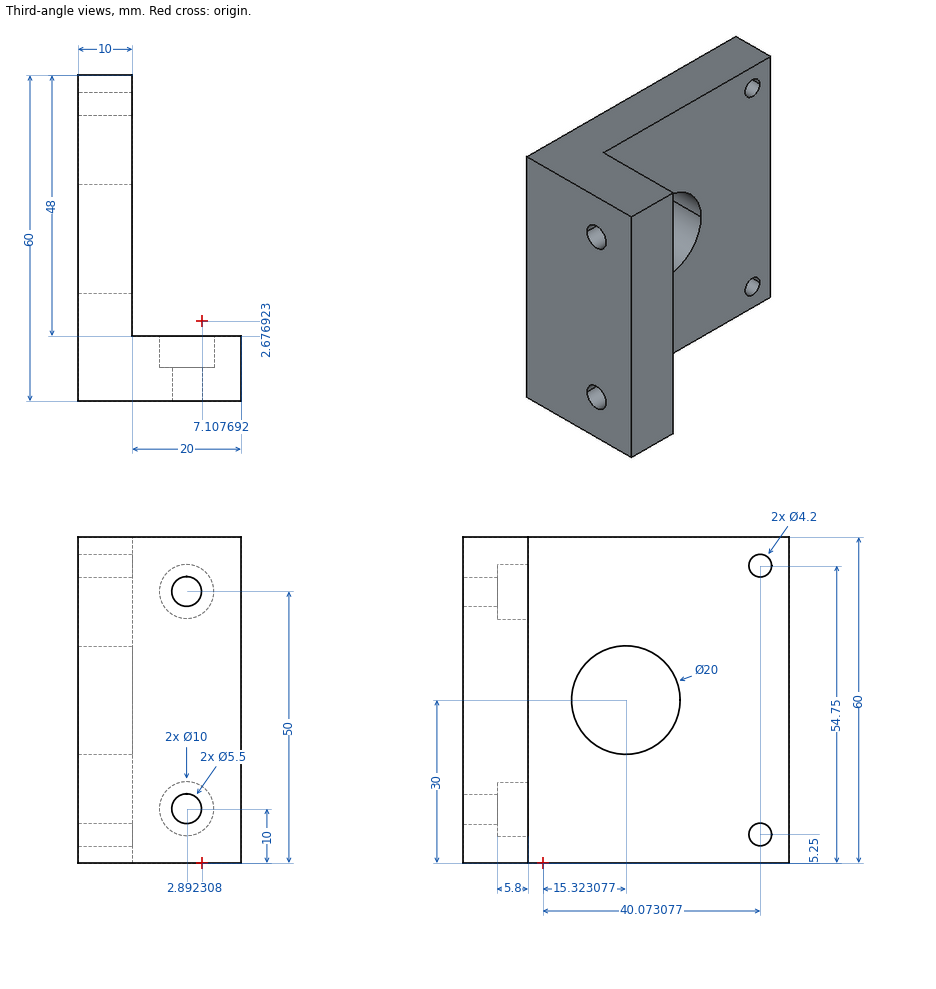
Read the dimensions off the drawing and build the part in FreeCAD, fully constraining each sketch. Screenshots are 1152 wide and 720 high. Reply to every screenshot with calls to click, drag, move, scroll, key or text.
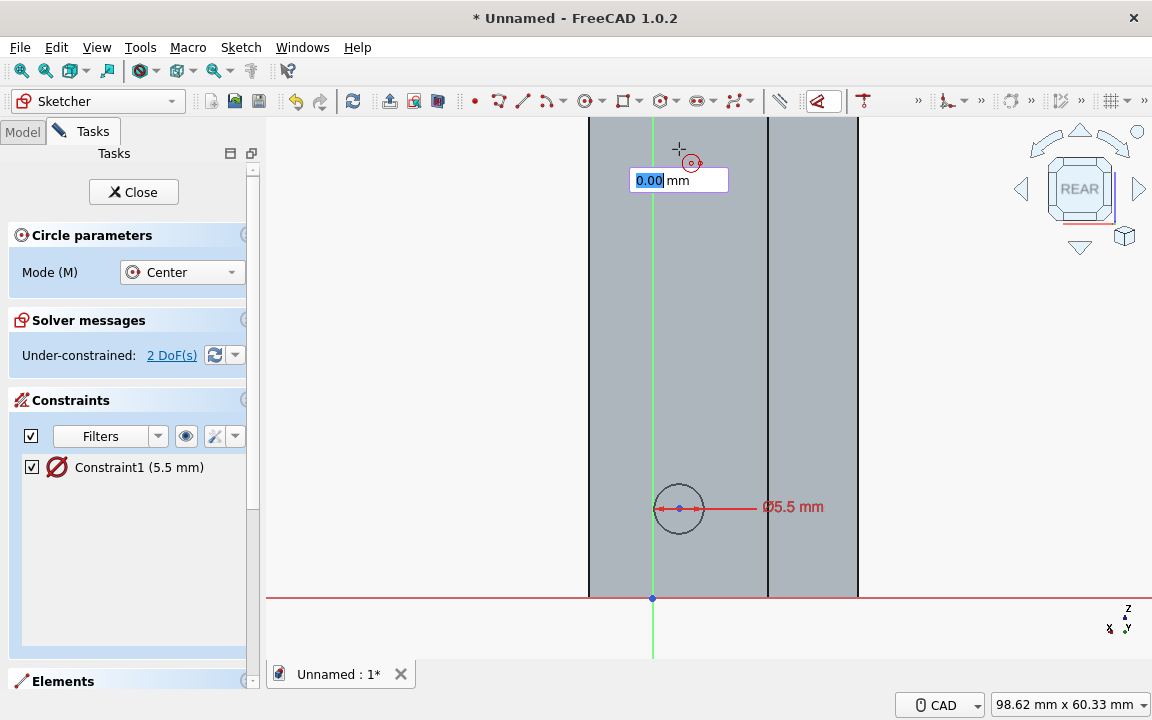
scroll(564, 443, down, 2)
move(653, 234)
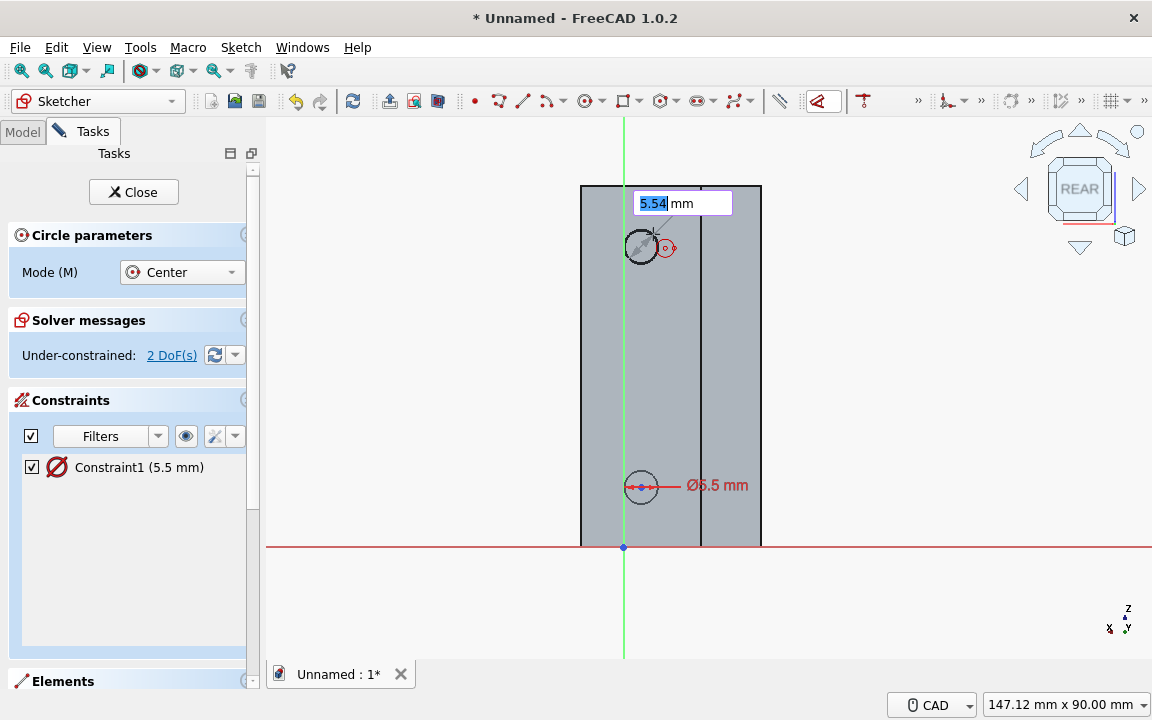
text(5.5)
key(Return)
key(Escape)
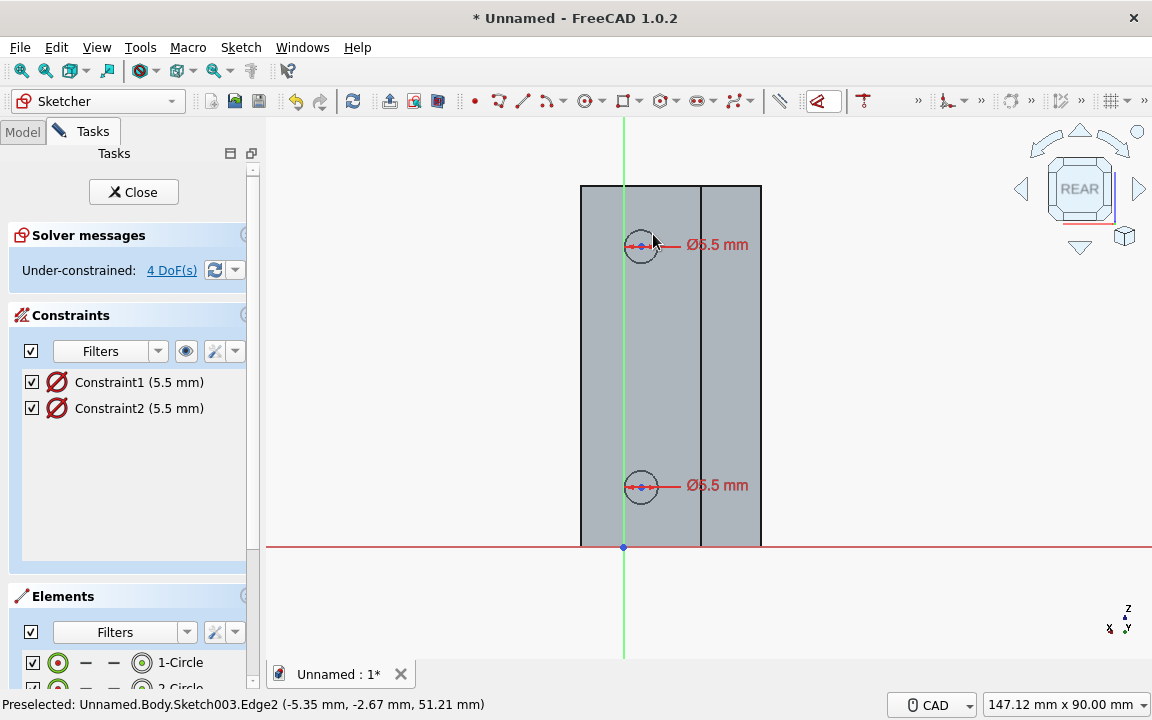
click(641, 487)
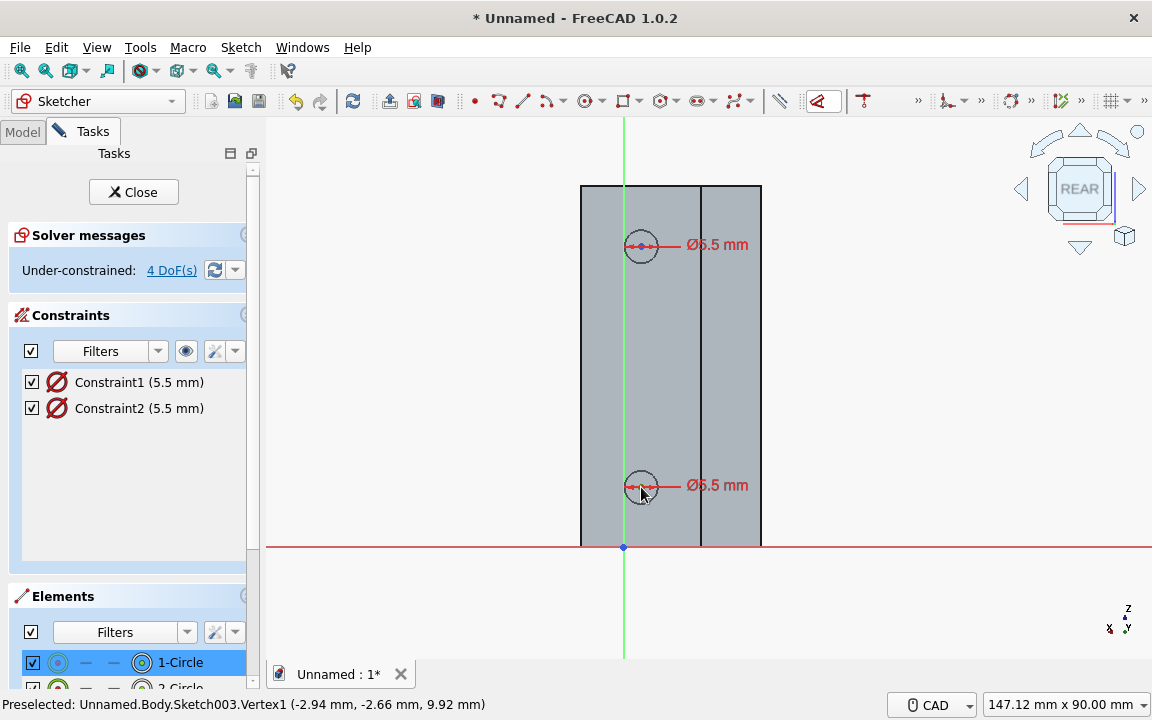
click(641, 247)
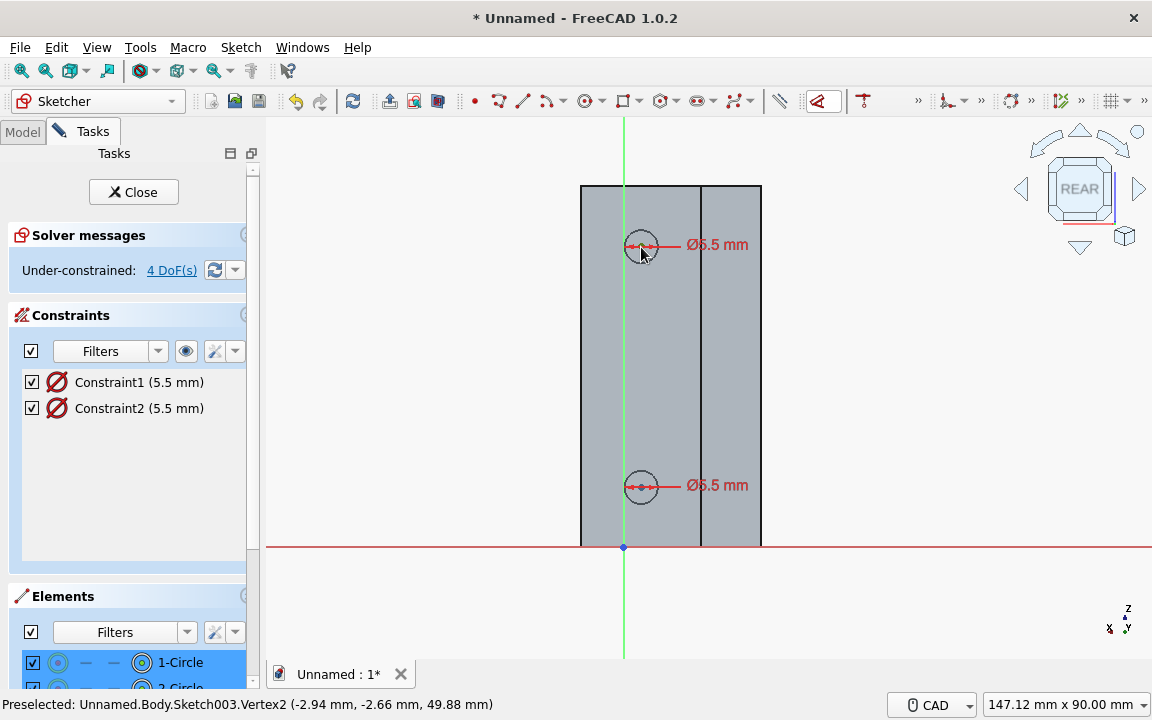
key(v)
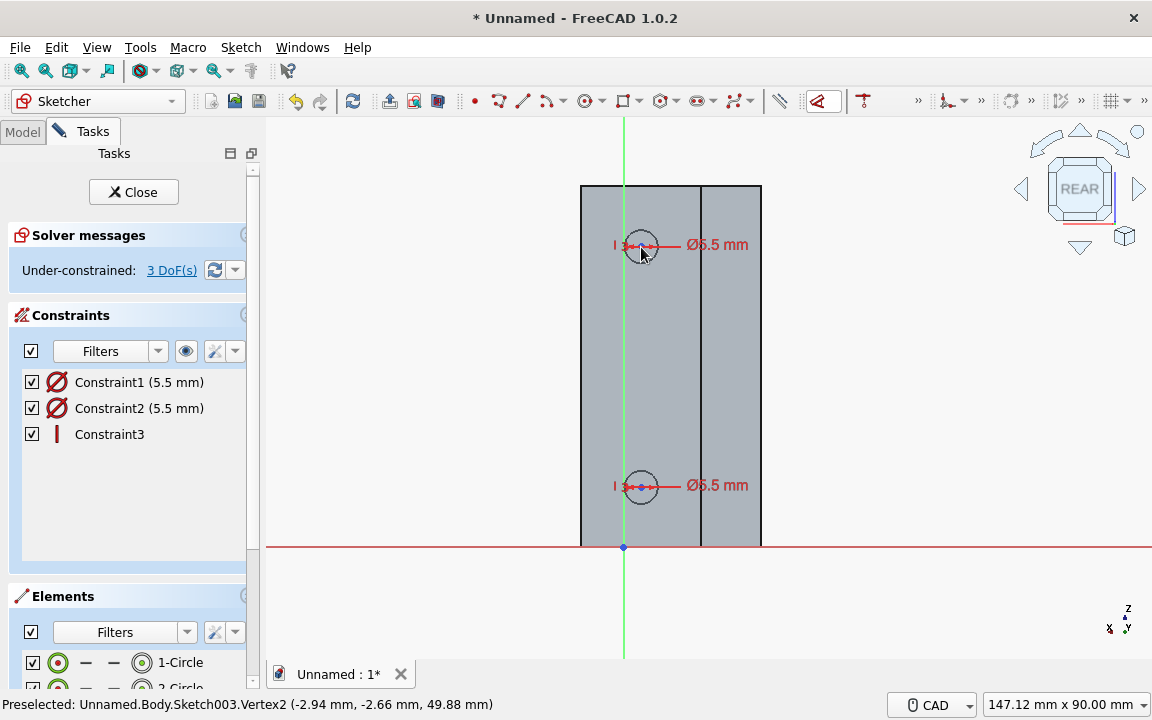
click(641, 487)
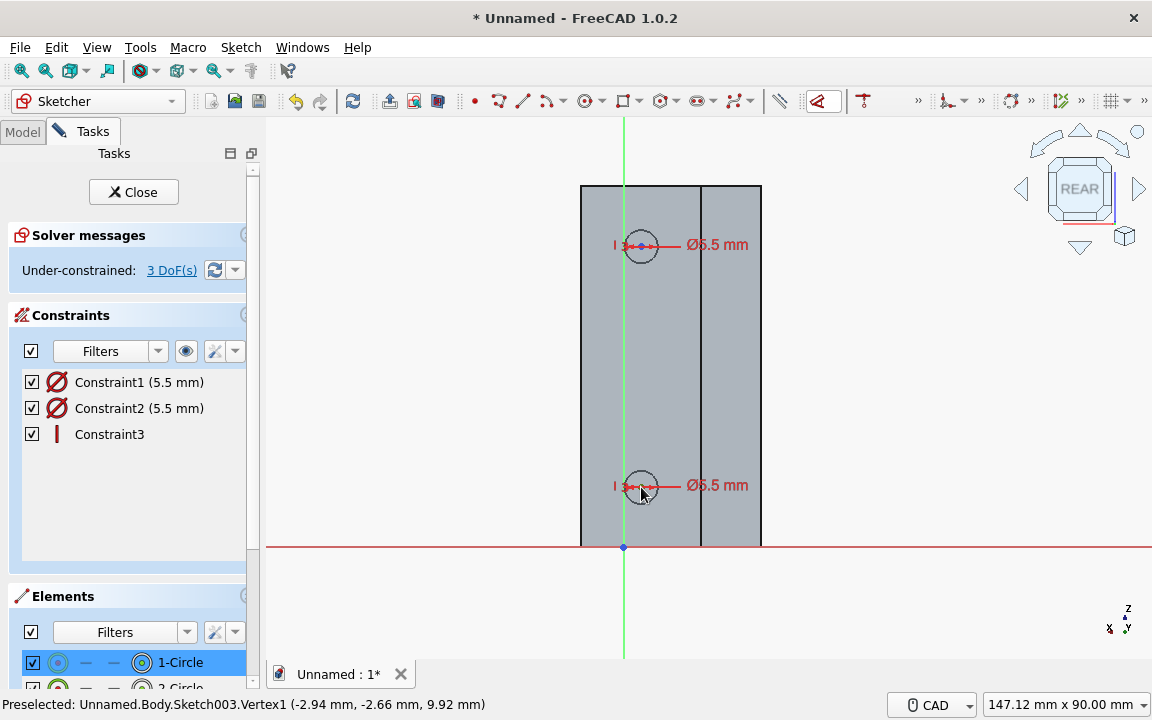
key(i)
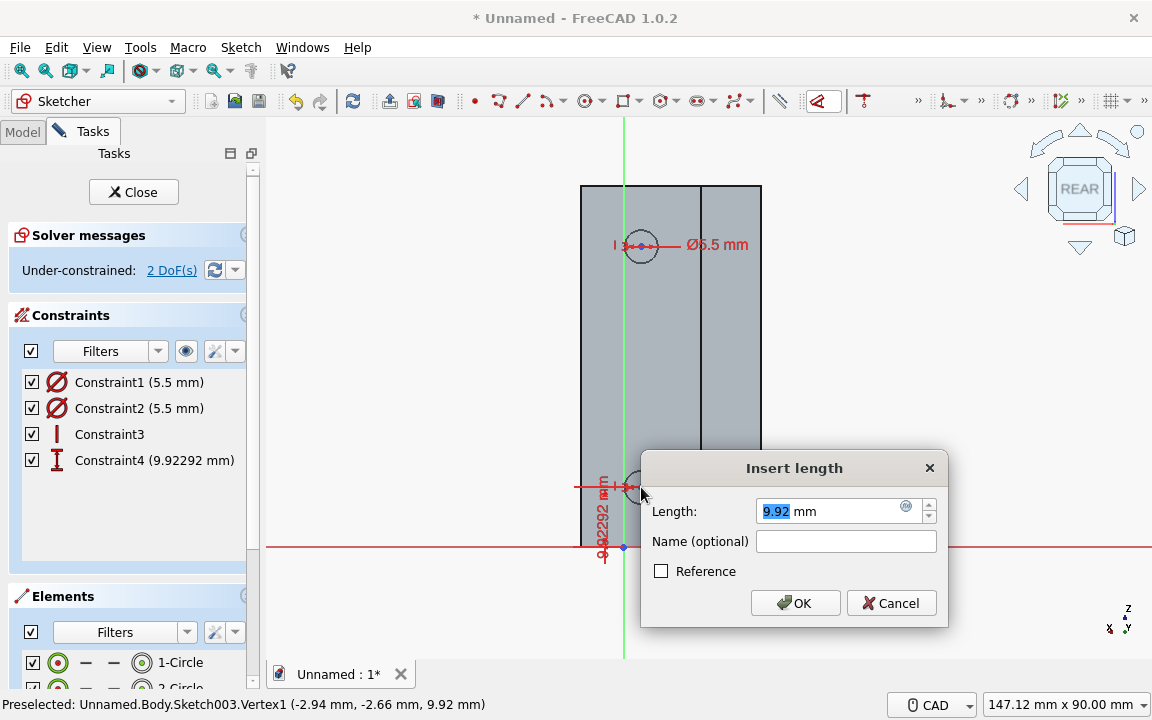
text(10)
key(Return)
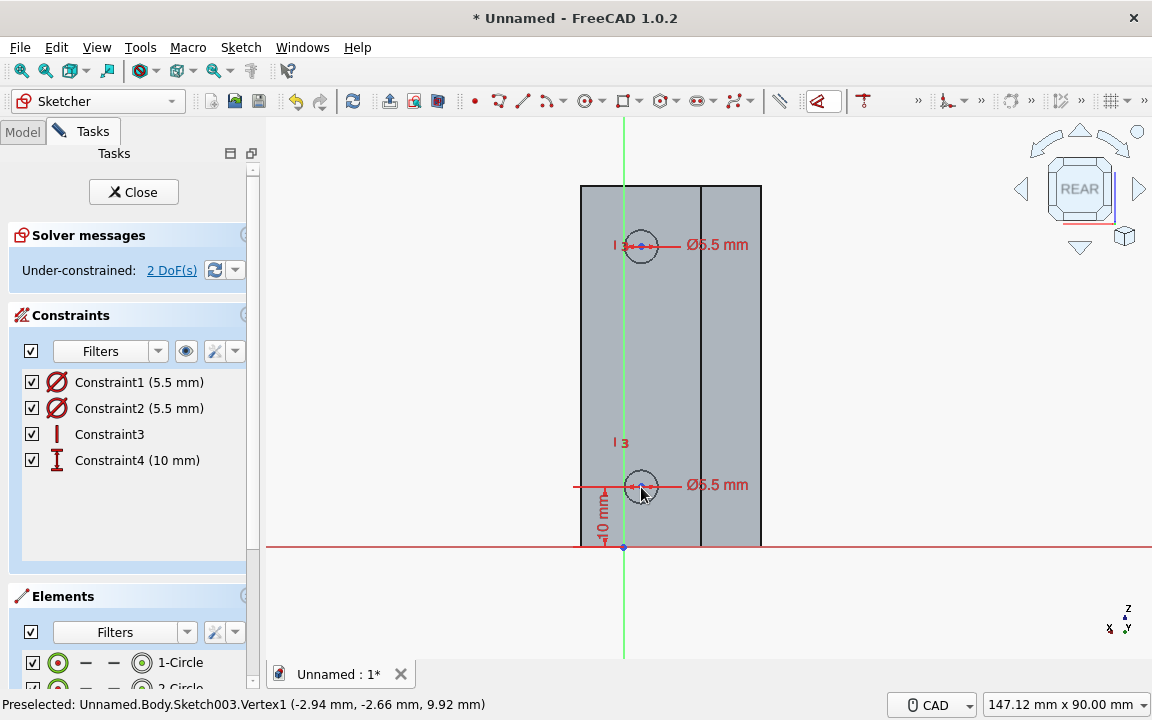
click(641, 247)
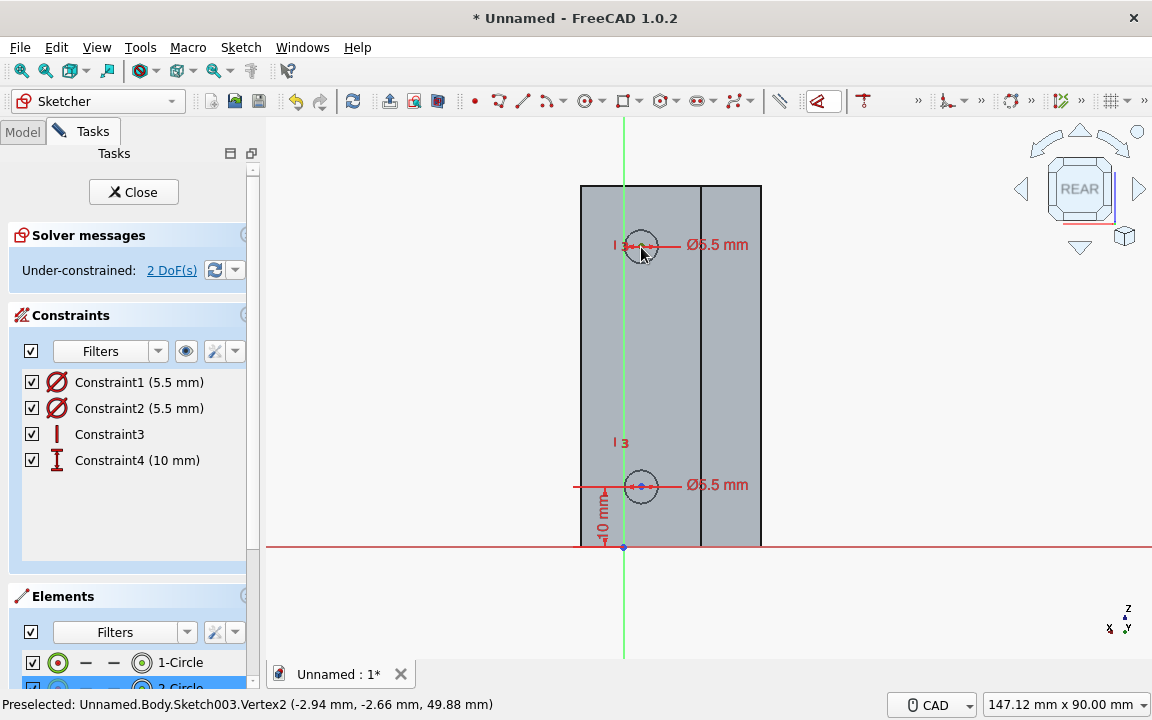
key(i)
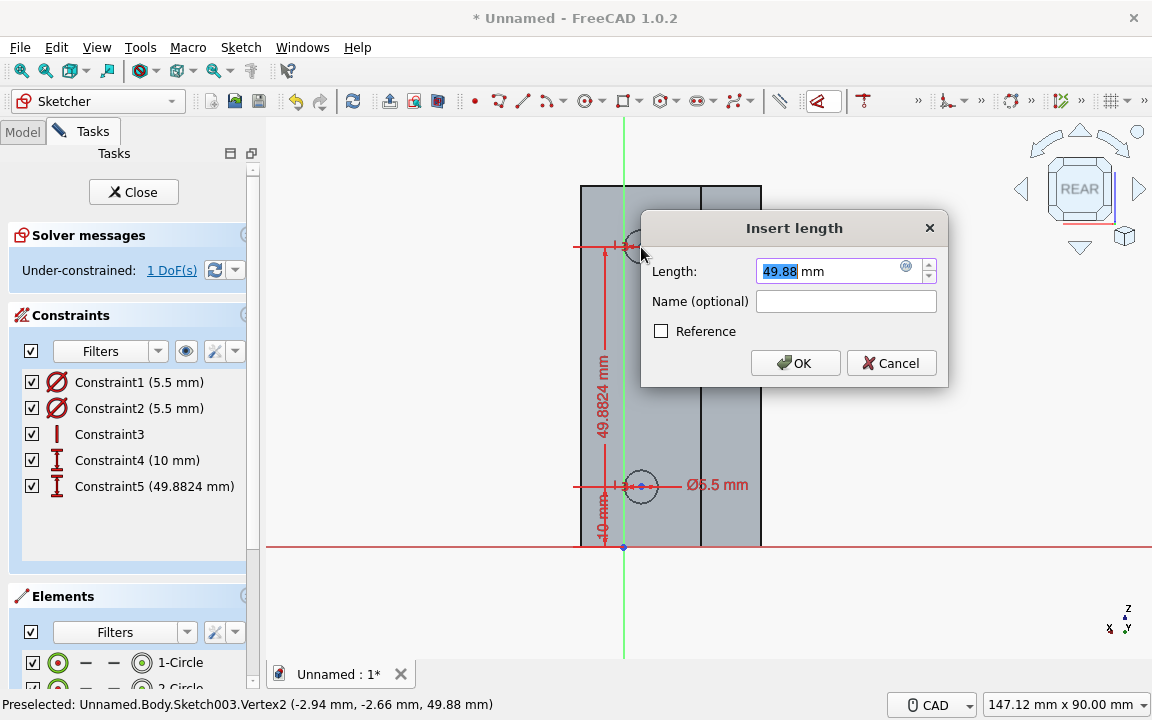
text(50)
key(Return)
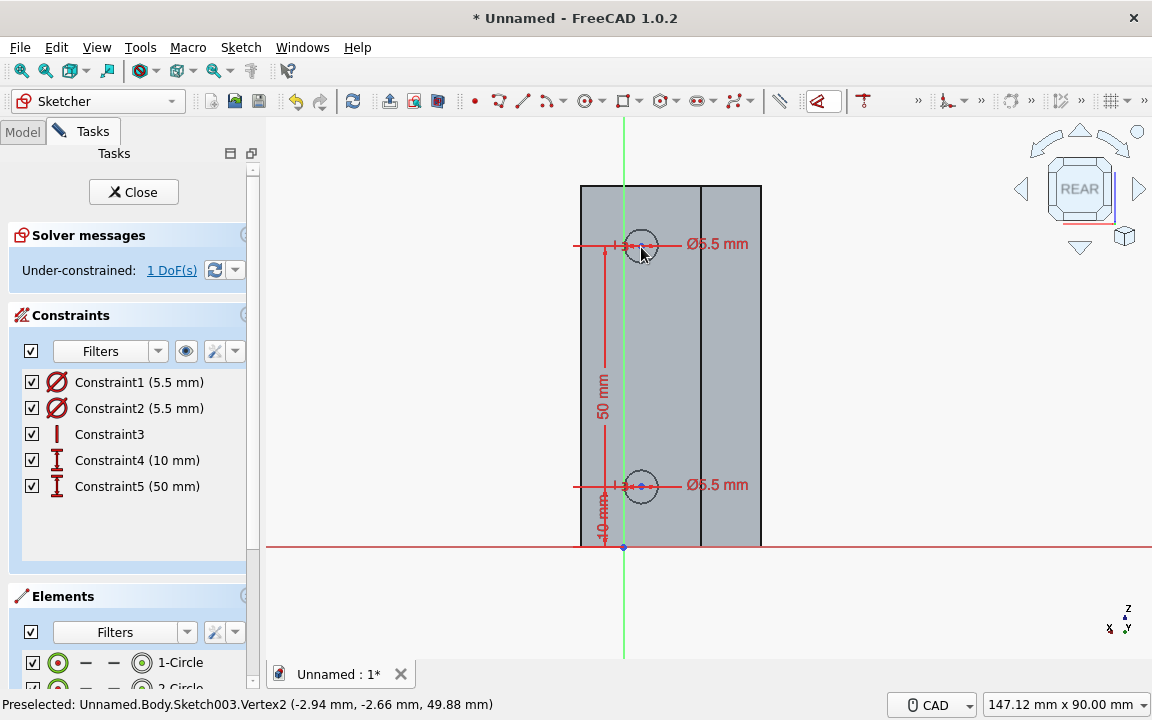
scroll(641, 487, up, 5)